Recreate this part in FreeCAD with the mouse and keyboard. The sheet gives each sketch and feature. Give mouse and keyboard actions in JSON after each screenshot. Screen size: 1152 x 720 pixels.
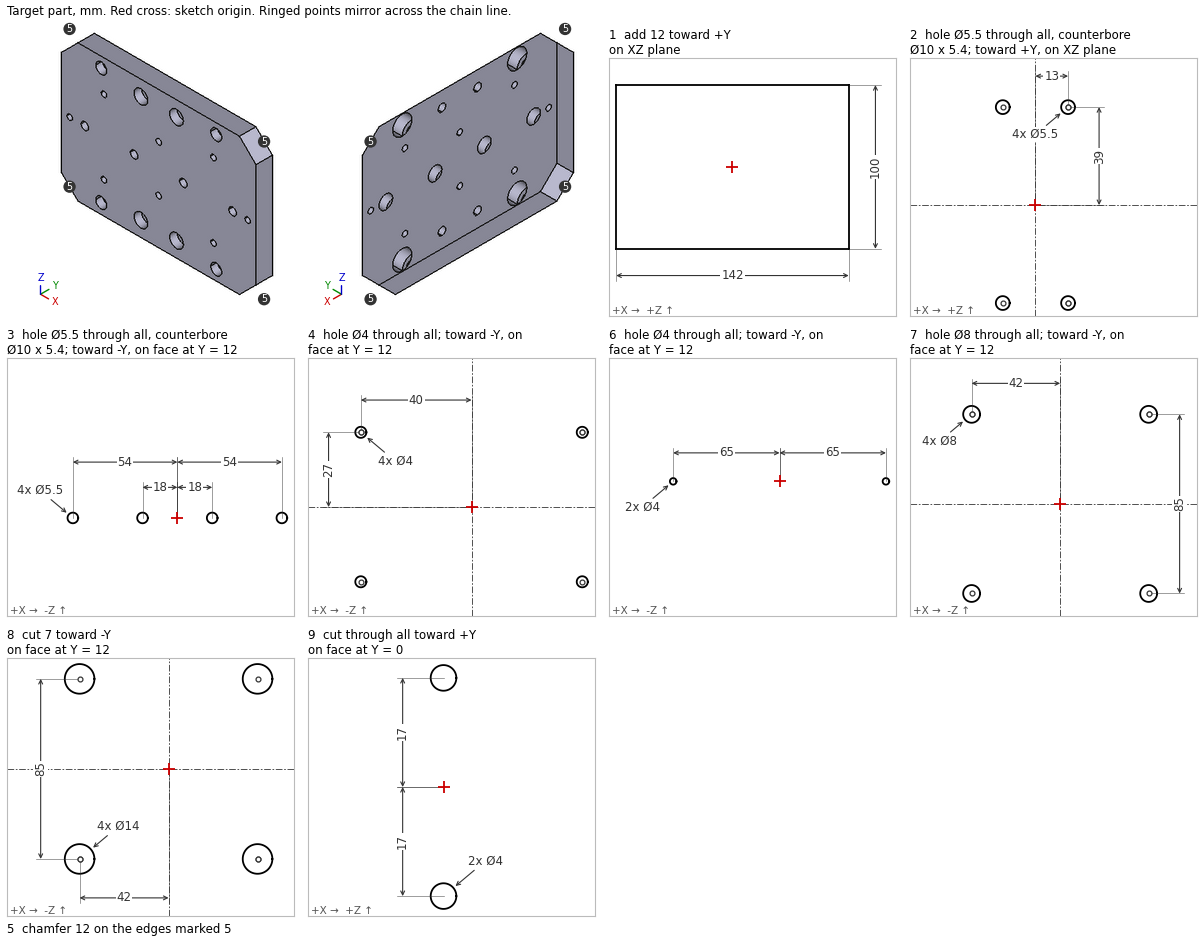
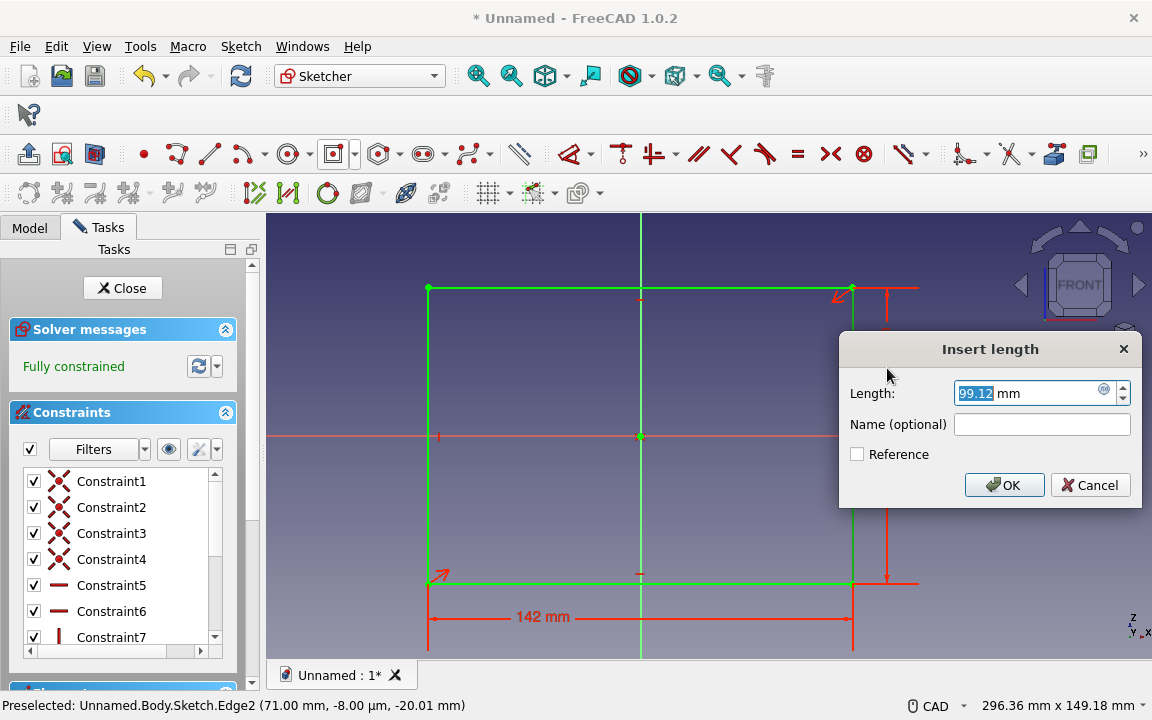
{"action": "type", "text": "100"}
{"action": "key", "text": "Return"}
{"action": "key", "text": "Escape"}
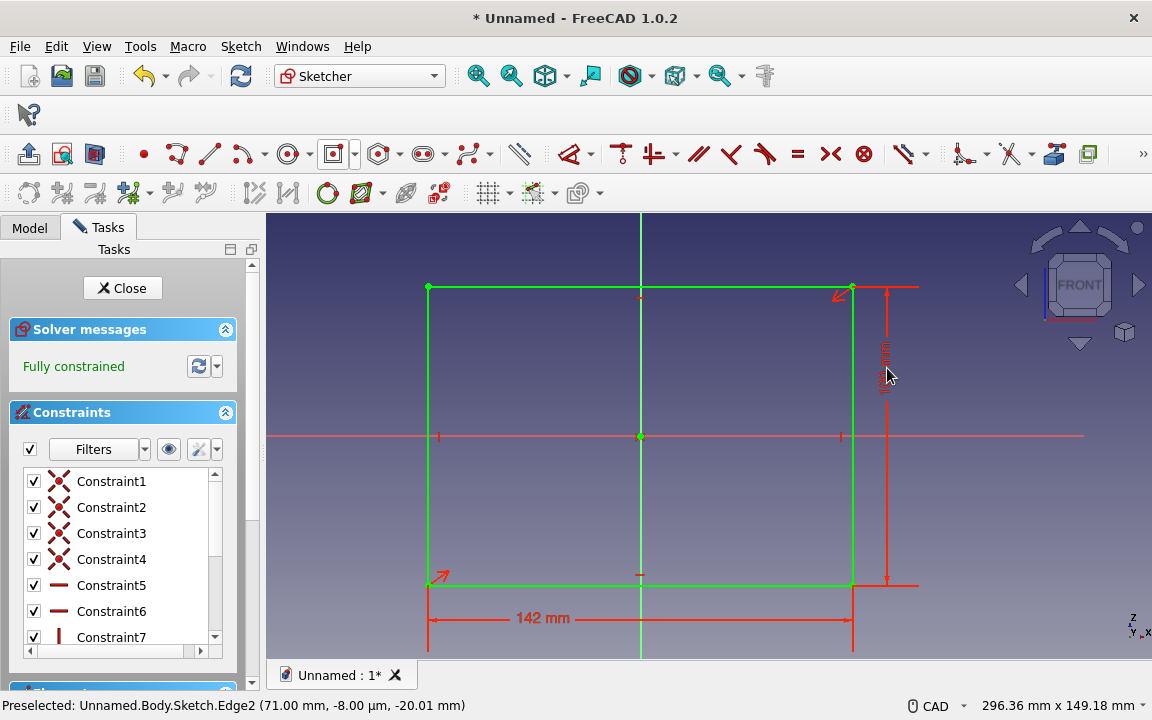
{"action": "left_click", "coordinate": [123, 288]}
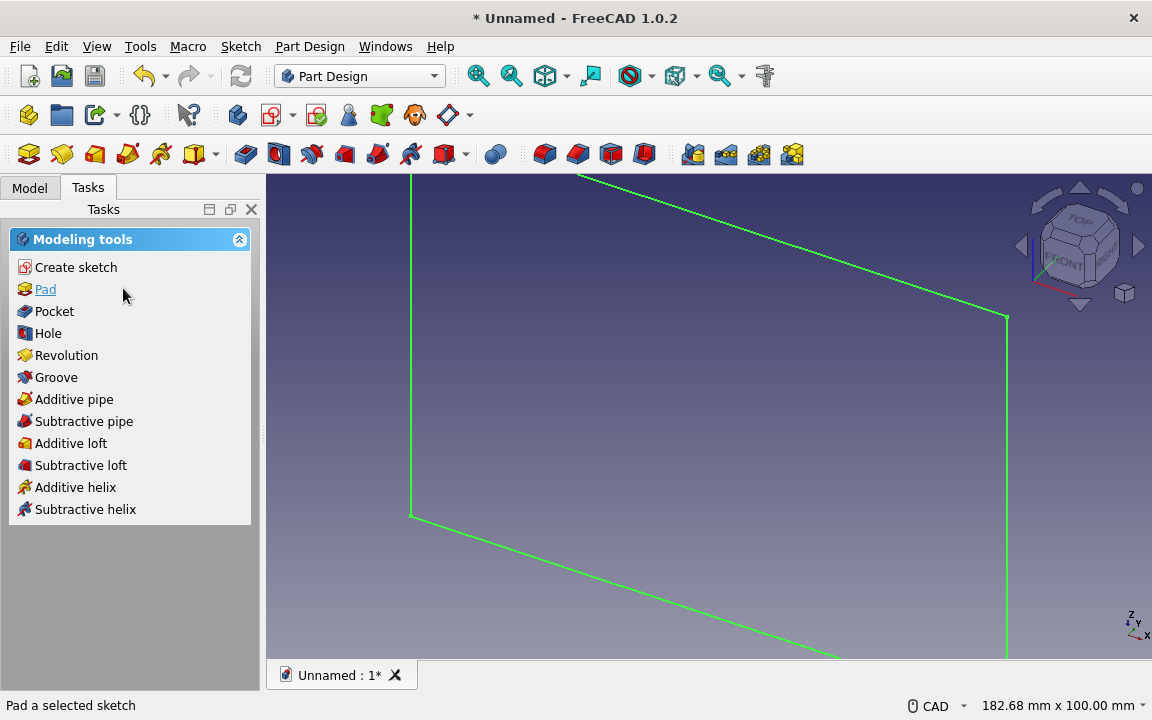
{"action": "left_click", "coordinate": [29, 154]}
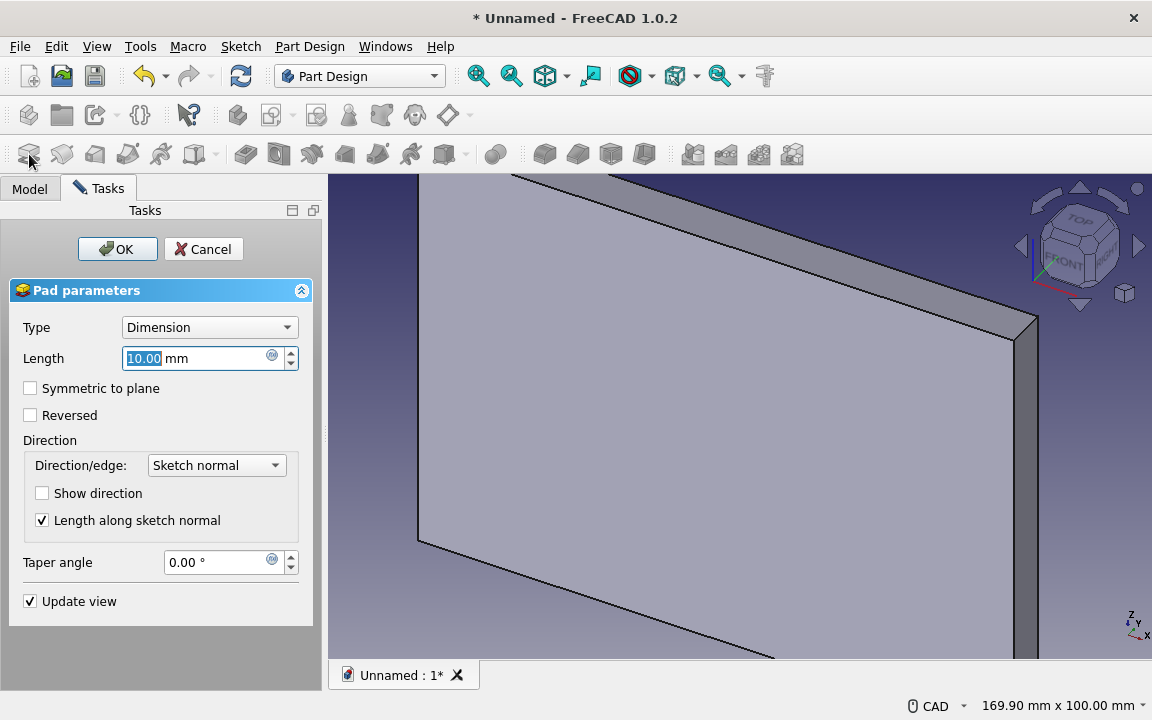
{"action": "type", "text": "12"}
{"action": "key", "text": "Tab"}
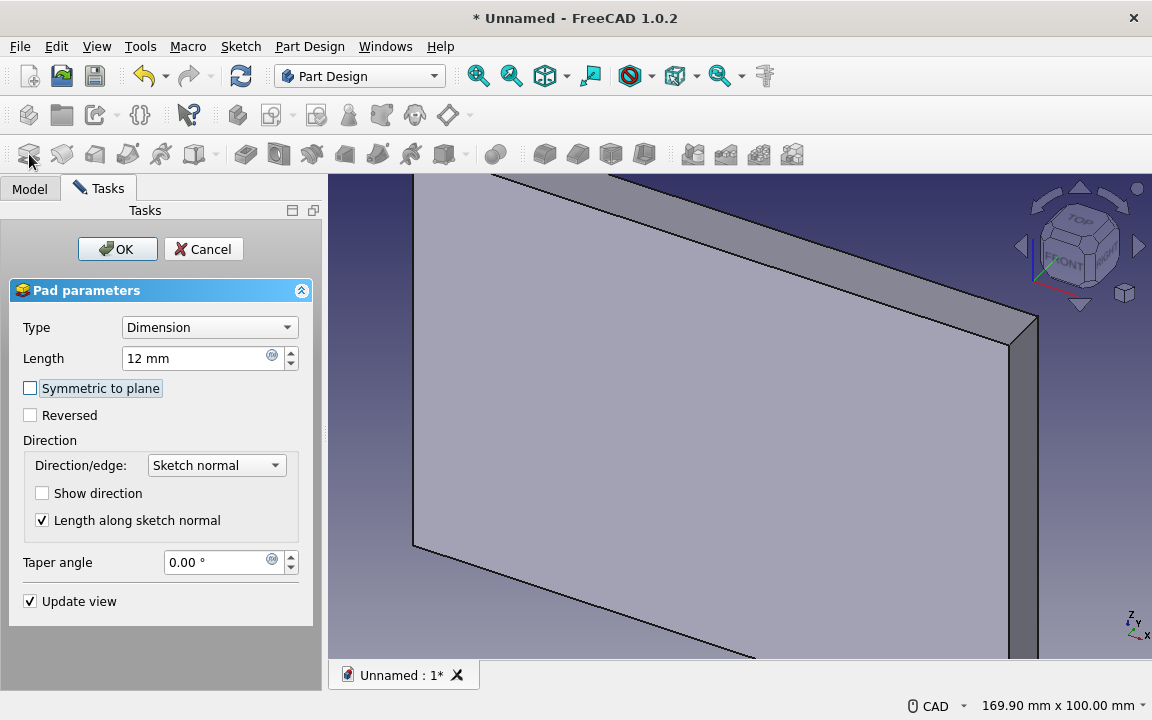
{"action": "left_click", "coordinate": [31, 415]}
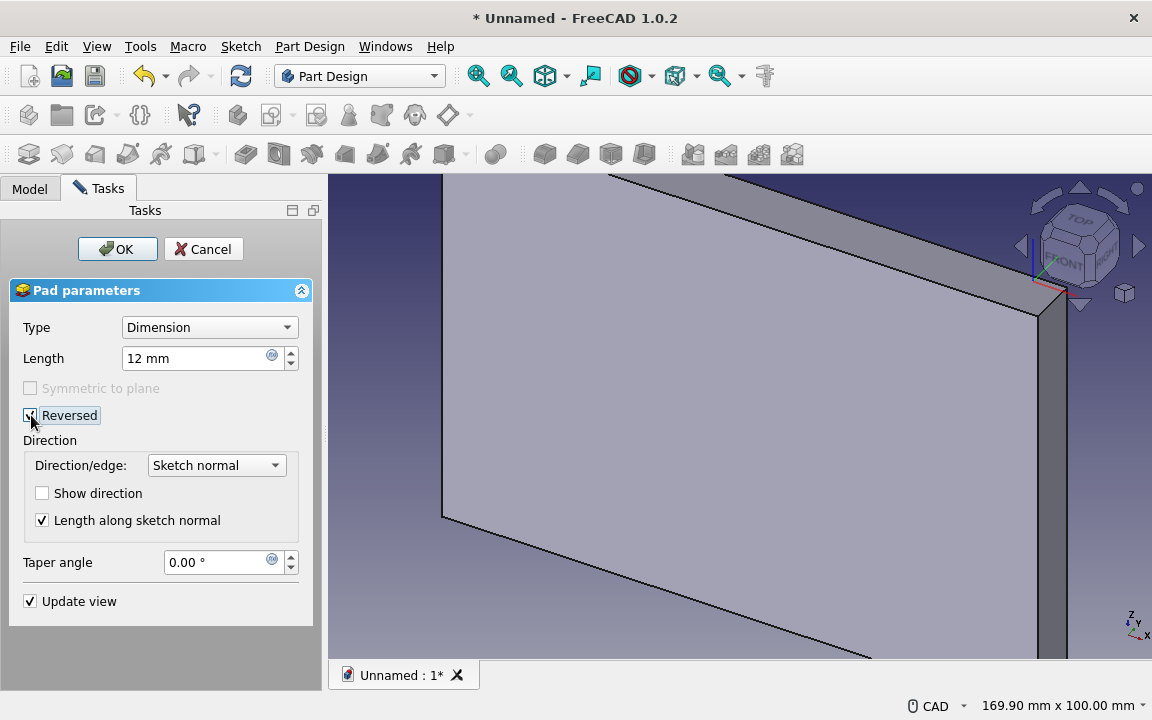
{"action": "left_click", "coordinate": [118, 249]}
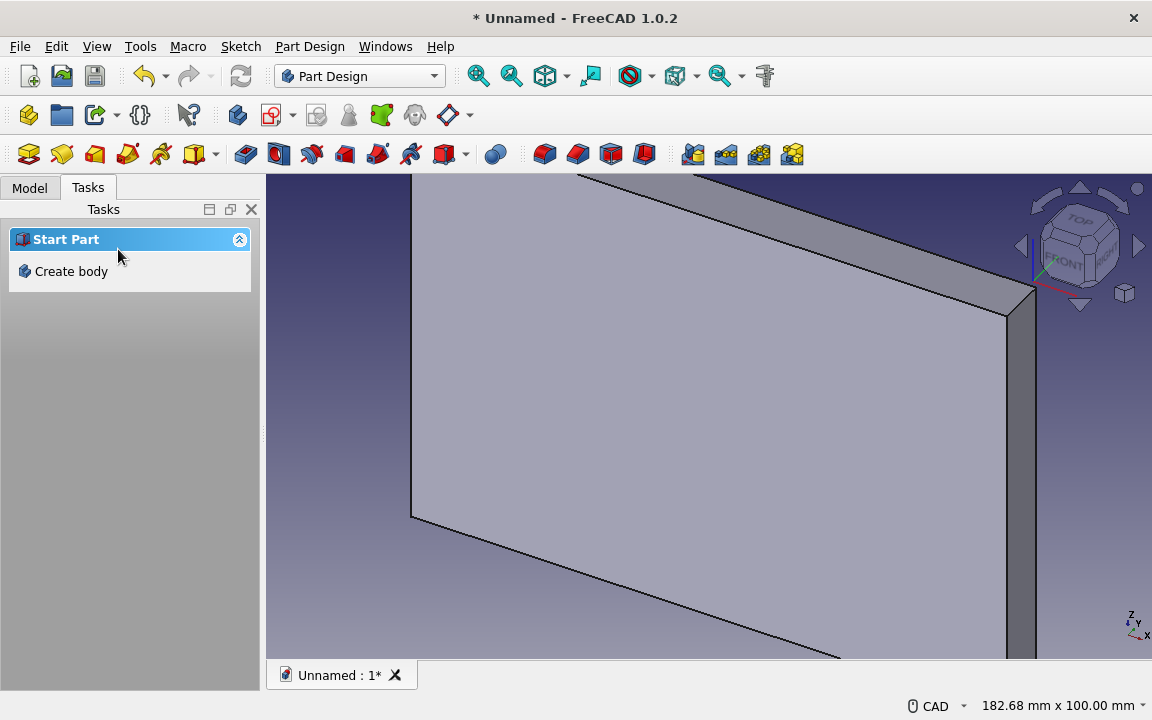
{"action": "left_click", "coordinate": [479, 76]}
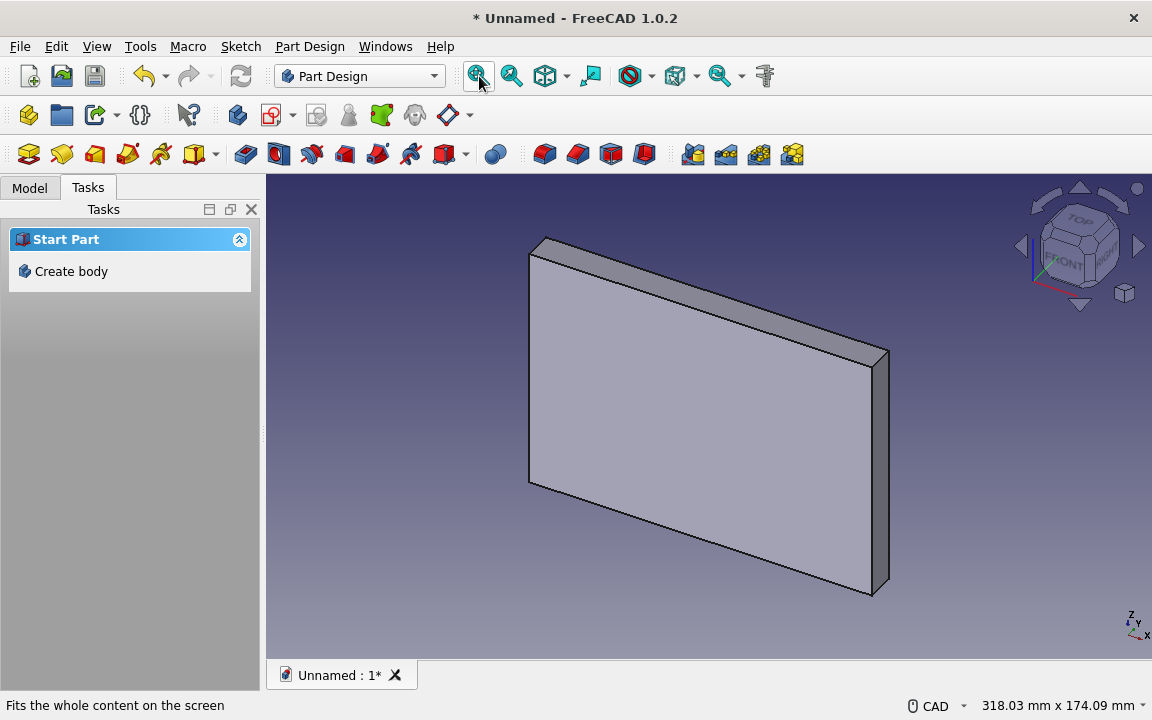
{"action": "left_click", "coordinate": [270, 116]}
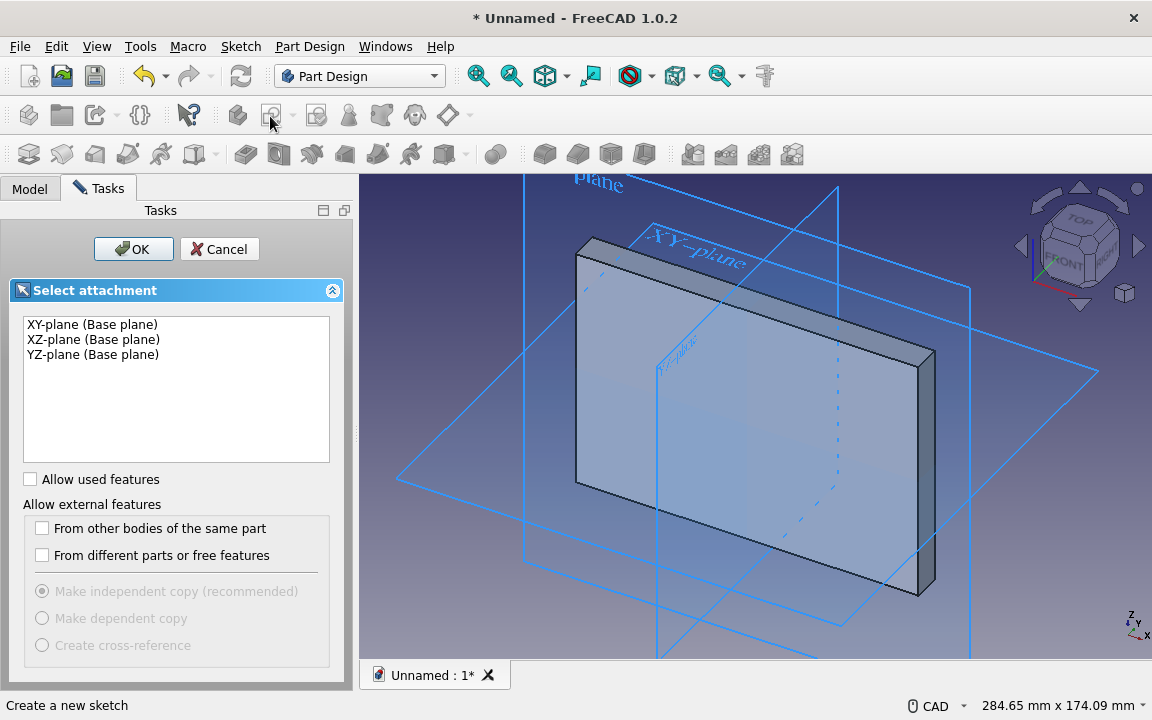
{"action": "left_click", "coordinate": [84, 340]}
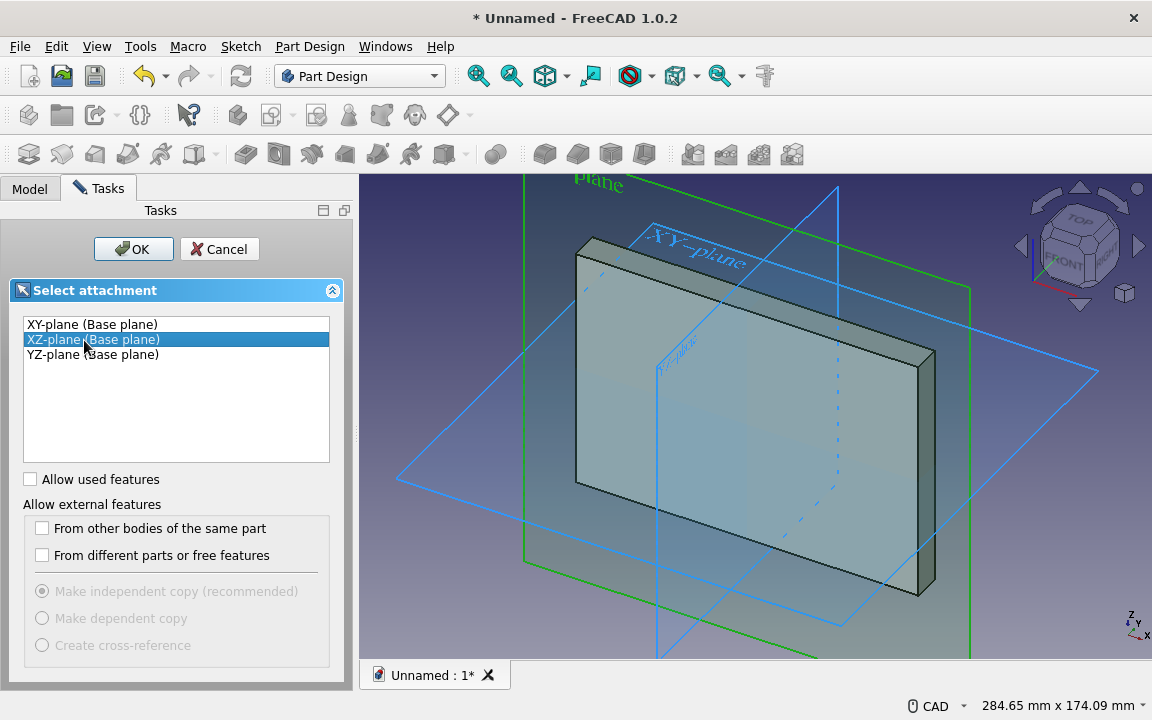
{"action": "left_click", "coordinate": [134, 249]}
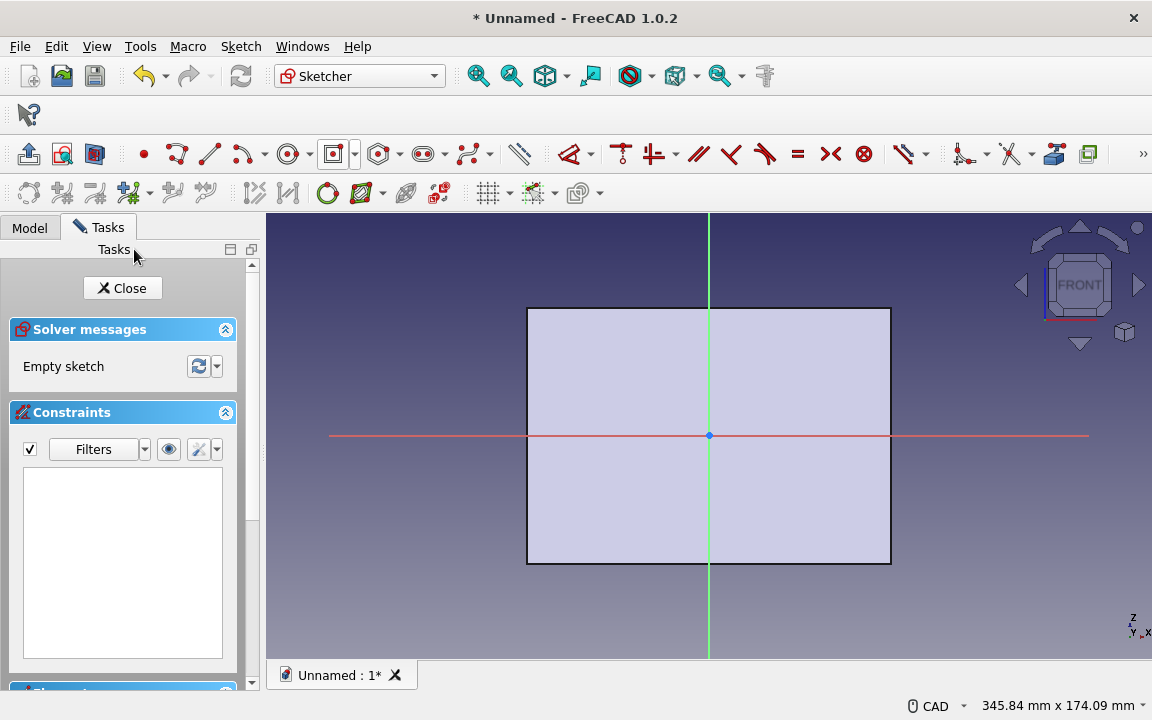
{"action": "left_click", "coordinate": [288, 154]}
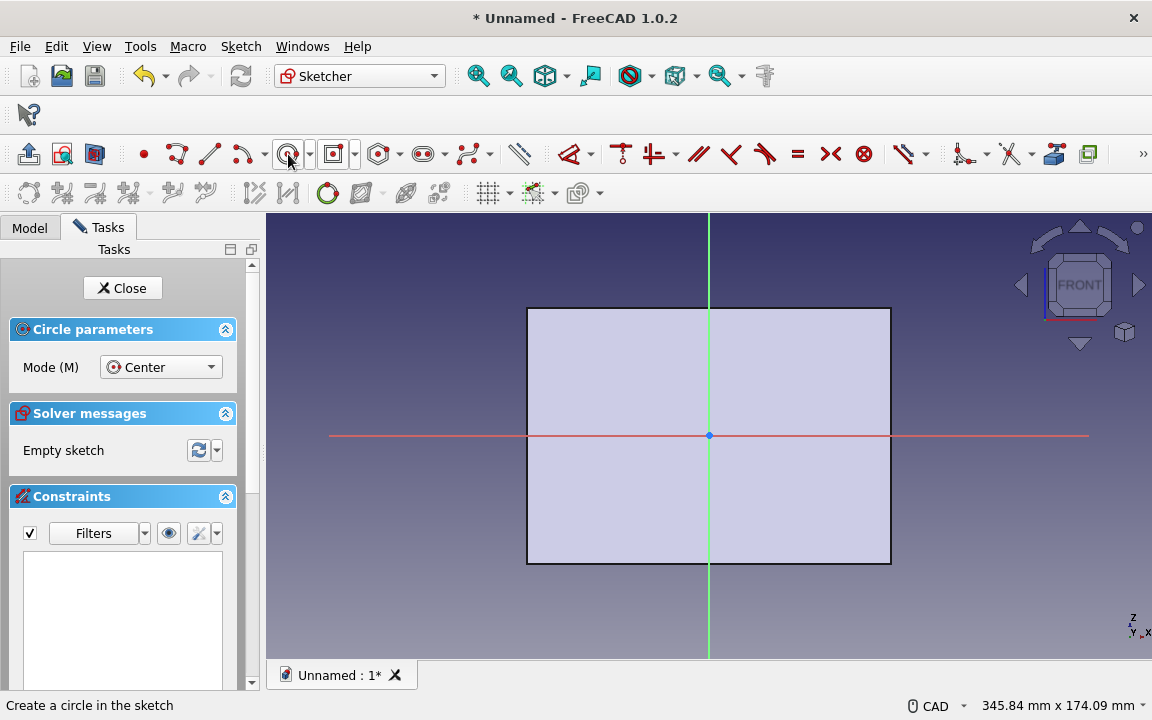
{"action": "scroll", "coordinate": [742, 336], "scroll_direction": "up", "scroll_amount": 6}